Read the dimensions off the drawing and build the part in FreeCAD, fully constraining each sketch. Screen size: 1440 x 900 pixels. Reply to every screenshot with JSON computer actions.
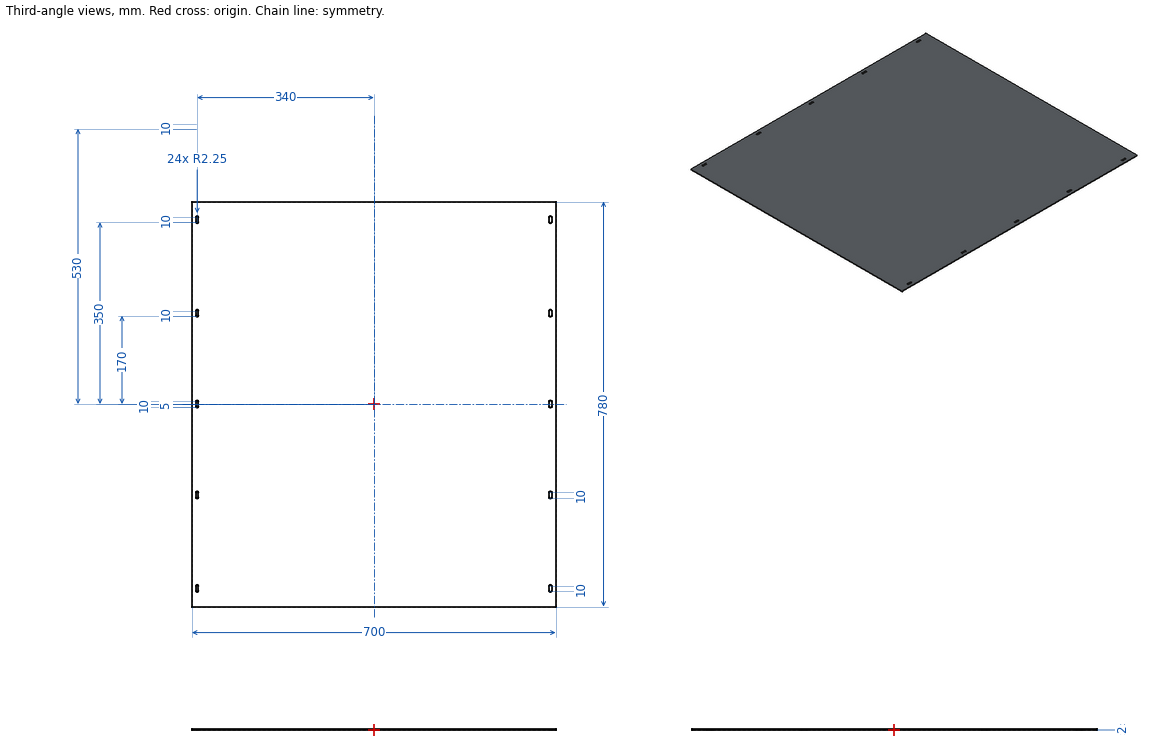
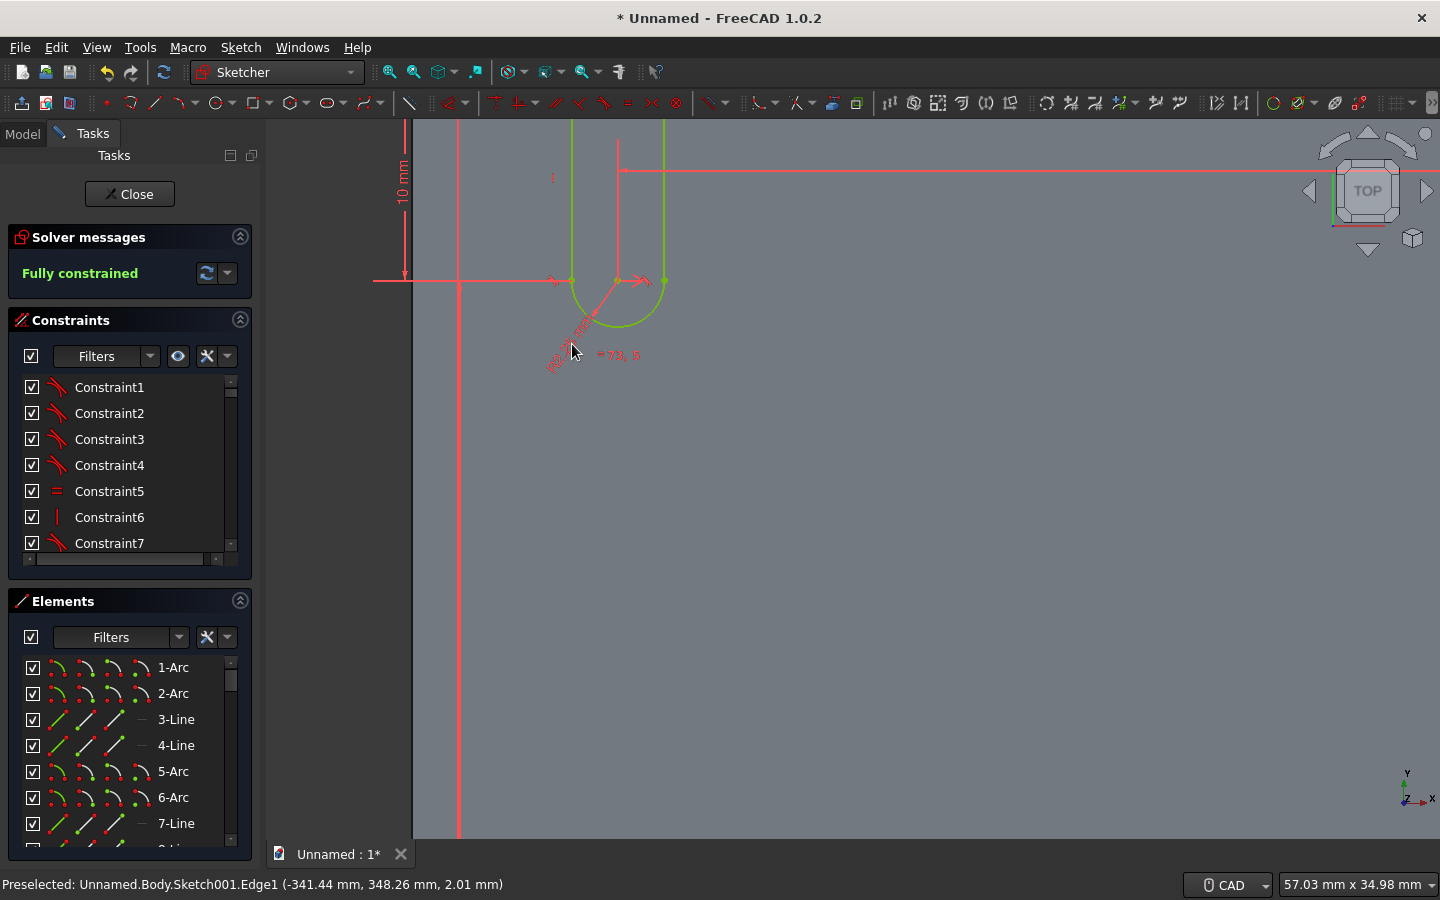
{"action": "left_click", "coordinate": [130, 194]}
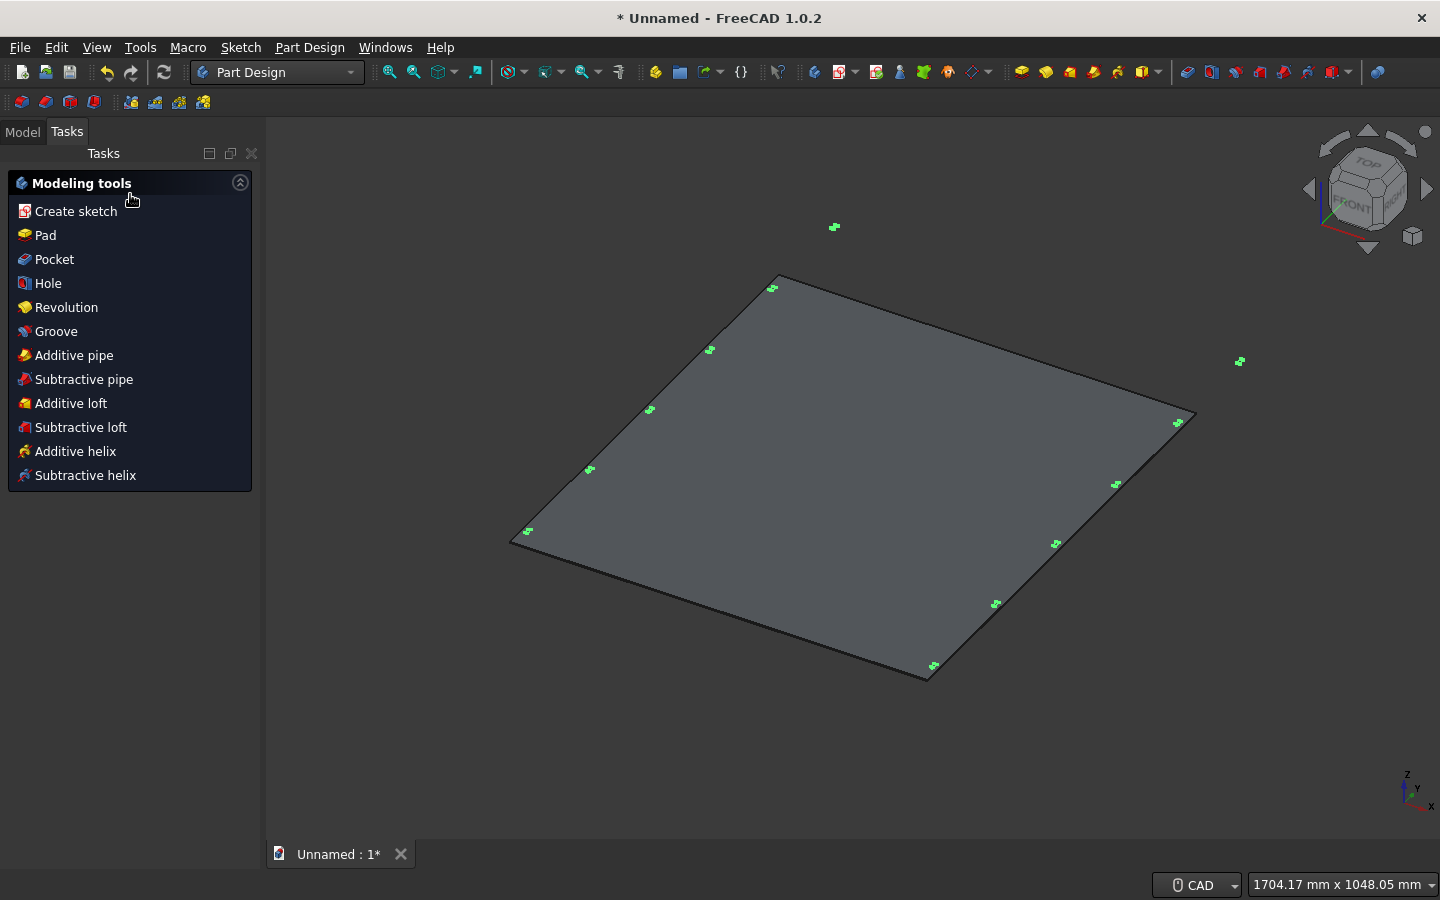
{"action": "left_click", "coordinate": [1188, 72]}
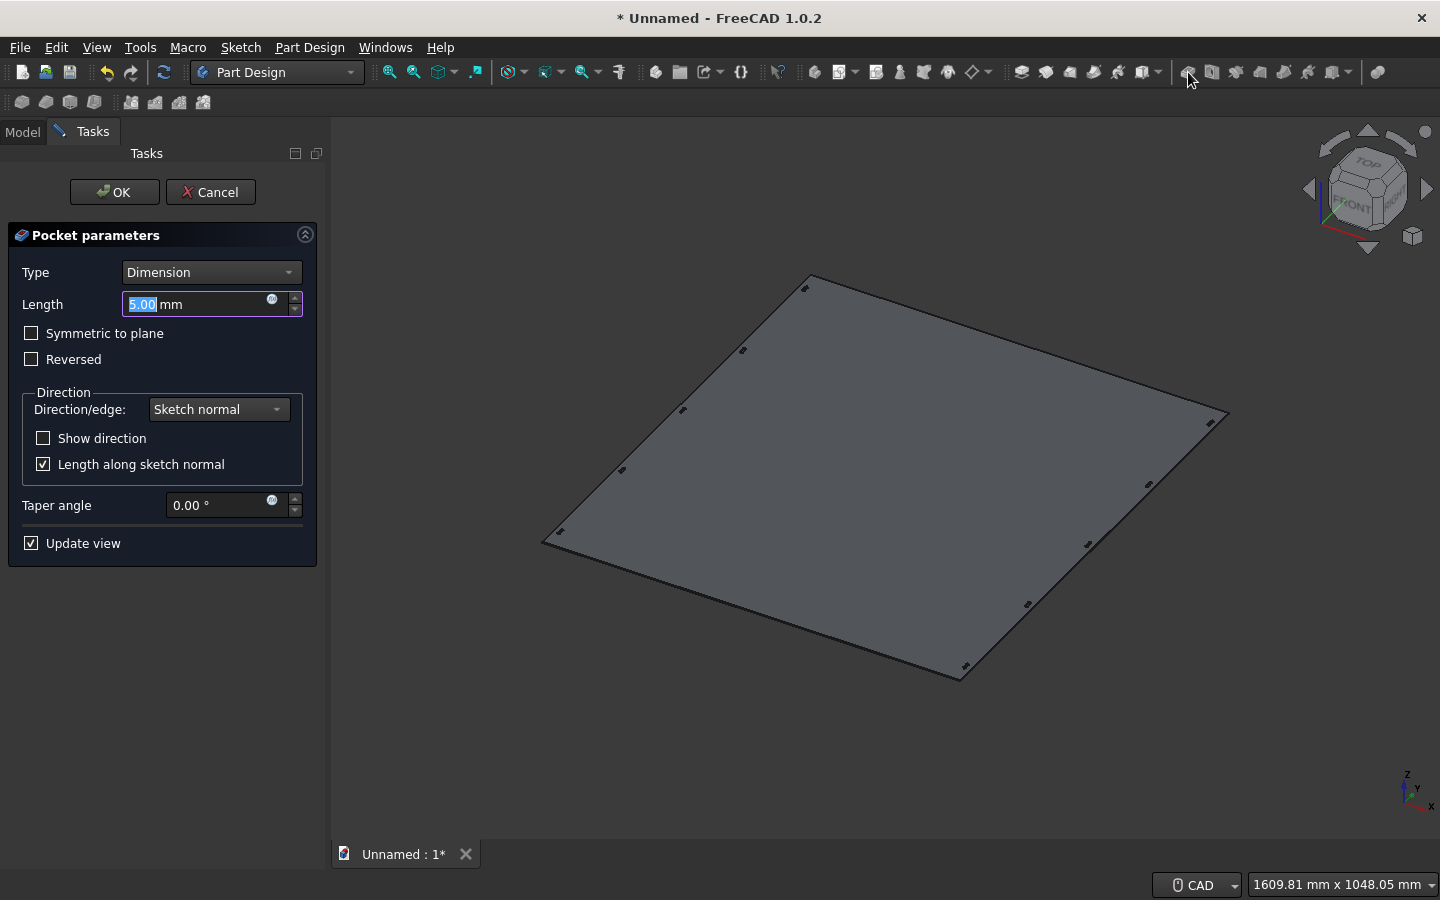
{"action": "type", "text": "10"}
{"action": "key", "text": "Tab"}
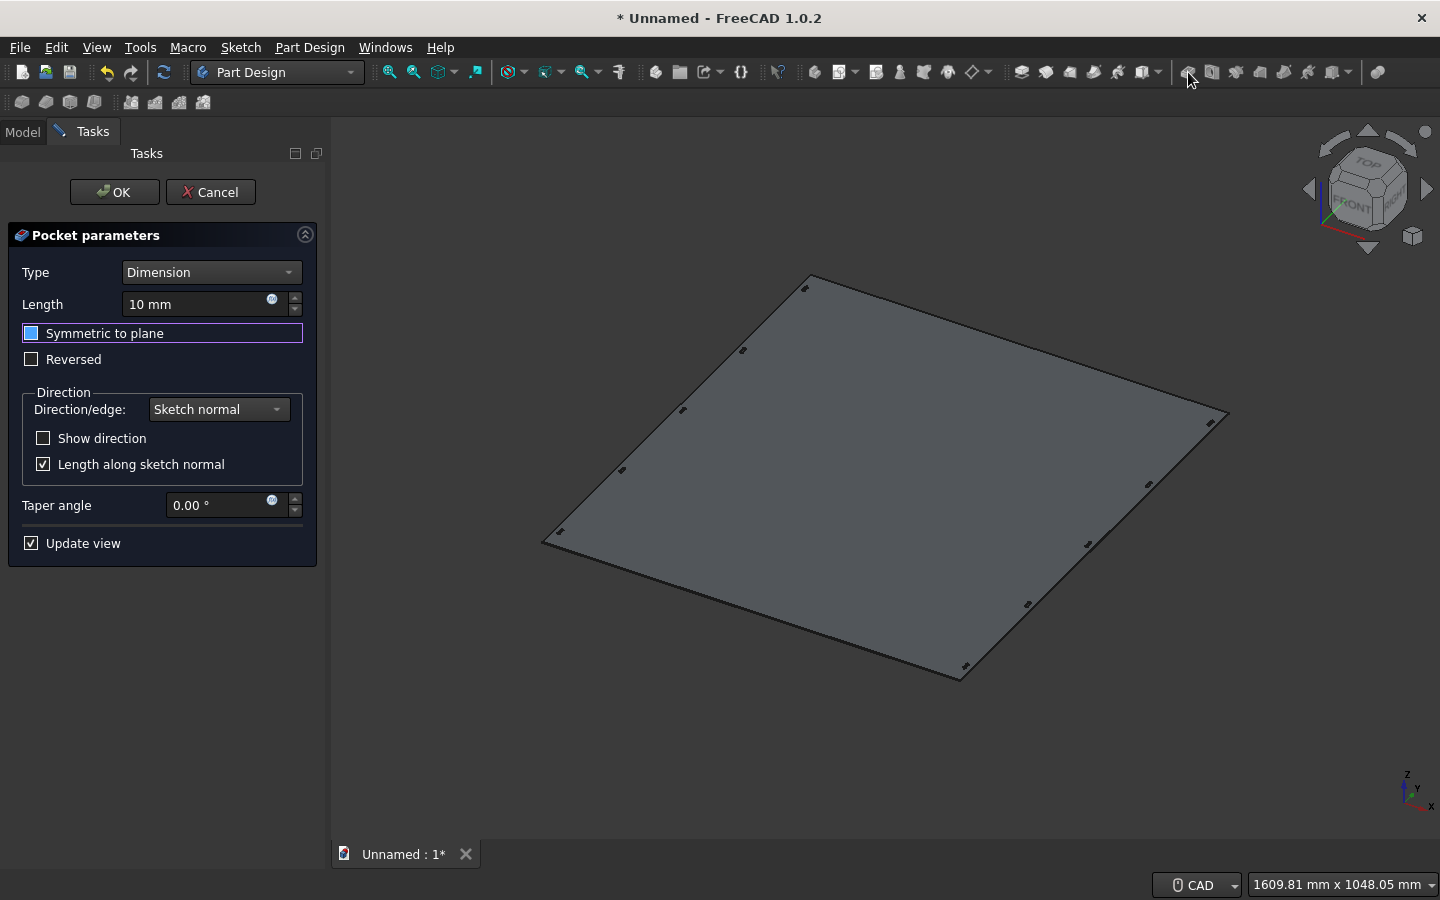
{"action": "left_click", "coordinate": [115, 192]}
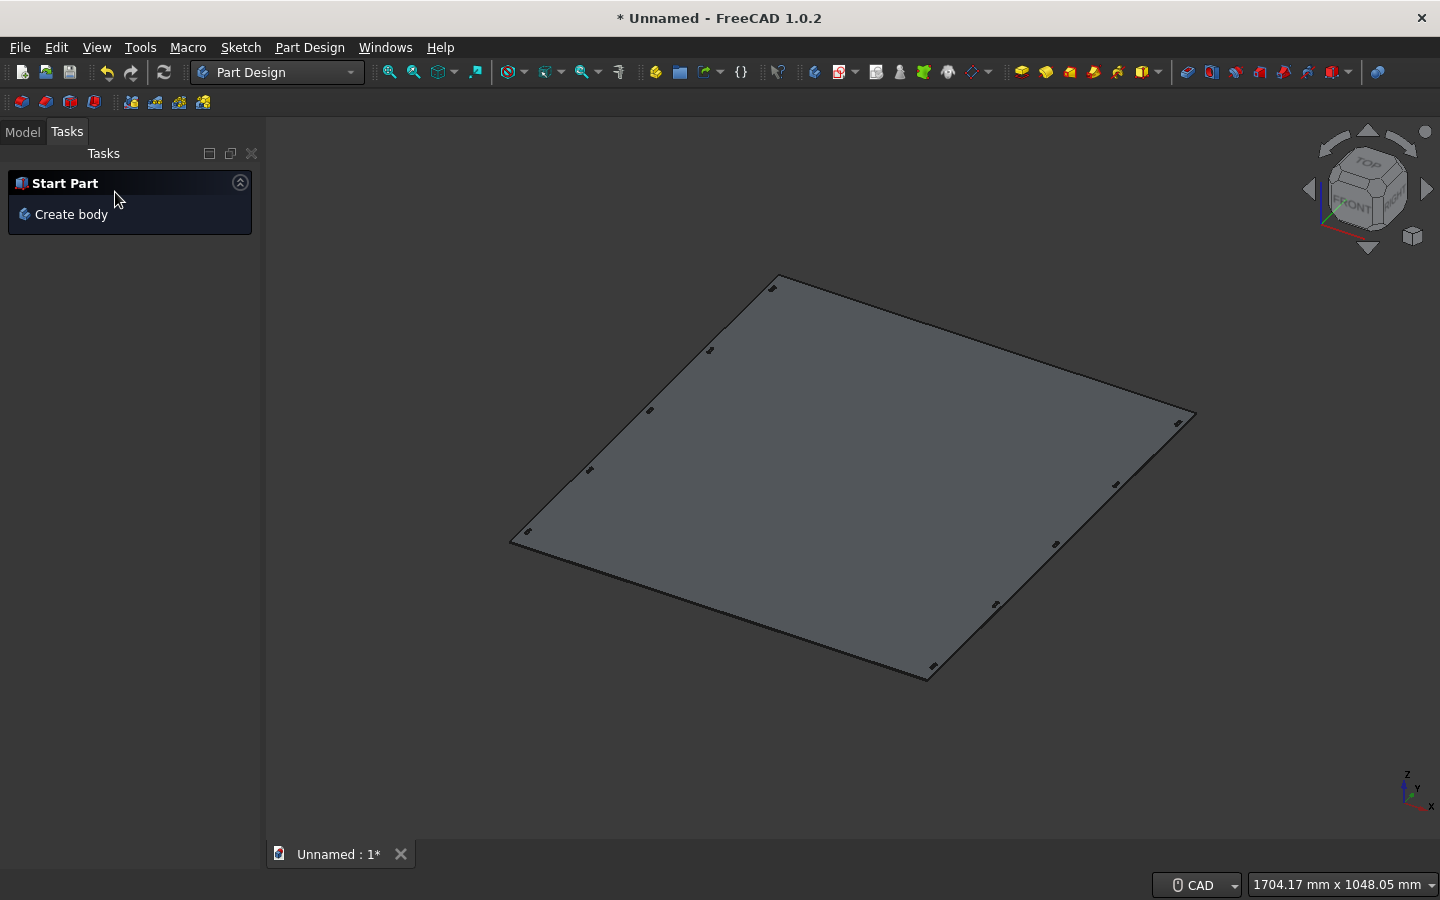
{"action": "key", "text": "0"}